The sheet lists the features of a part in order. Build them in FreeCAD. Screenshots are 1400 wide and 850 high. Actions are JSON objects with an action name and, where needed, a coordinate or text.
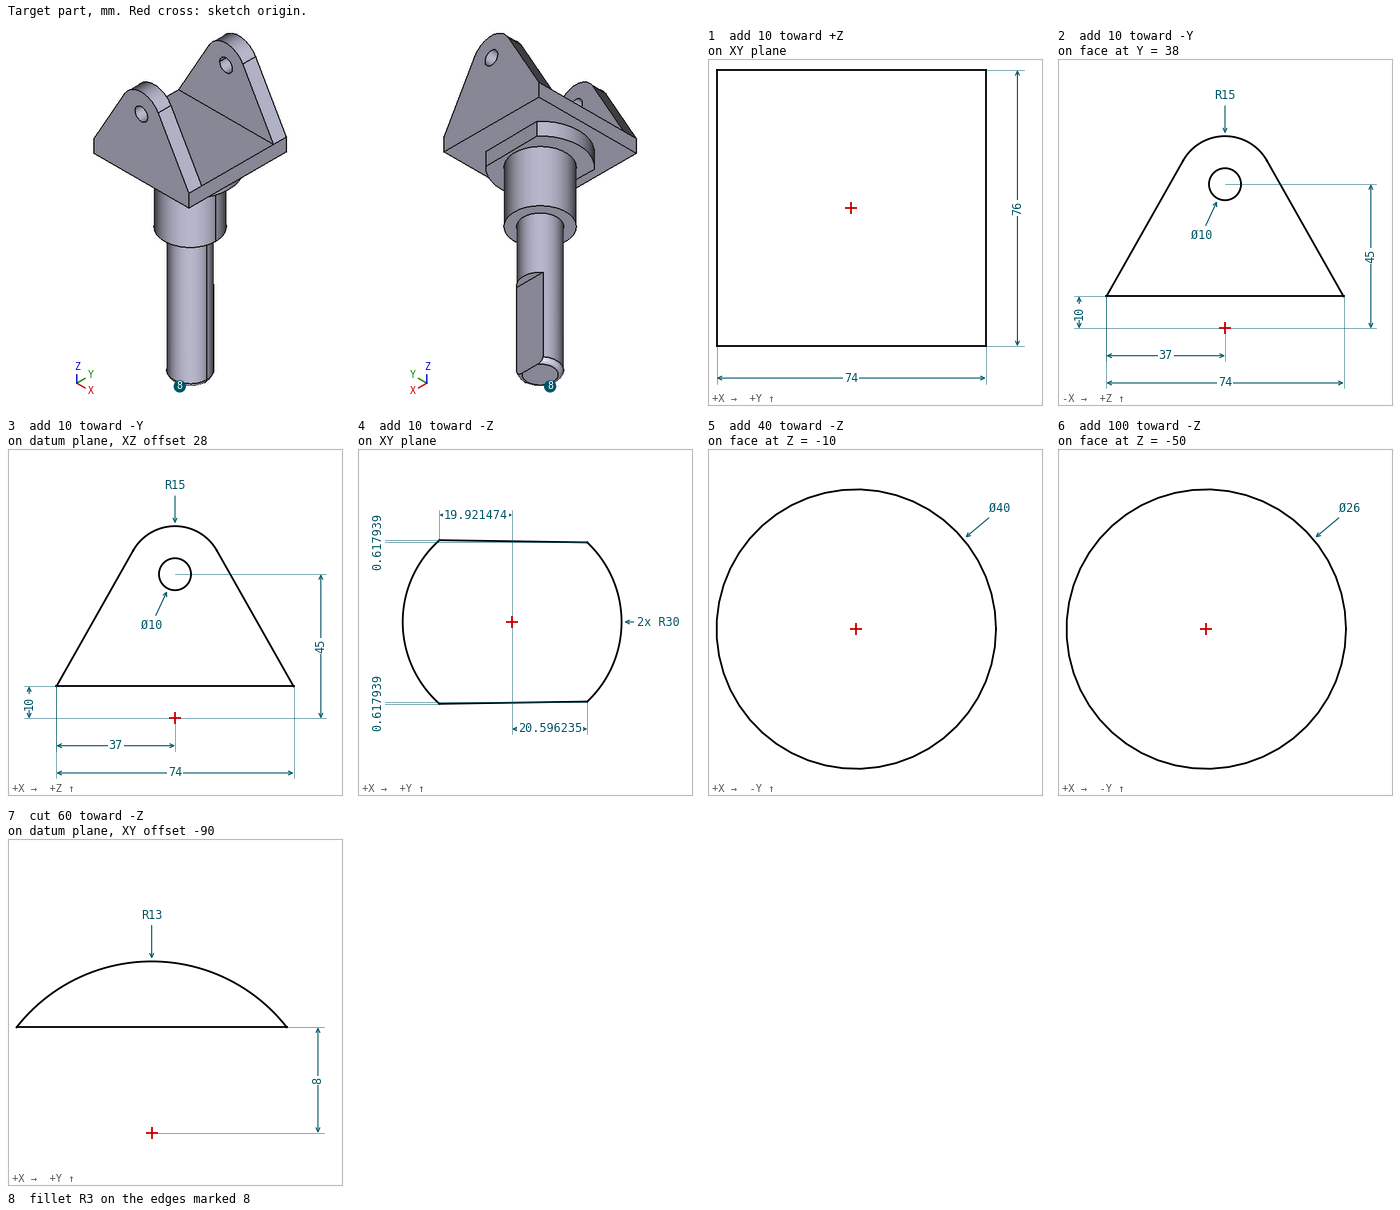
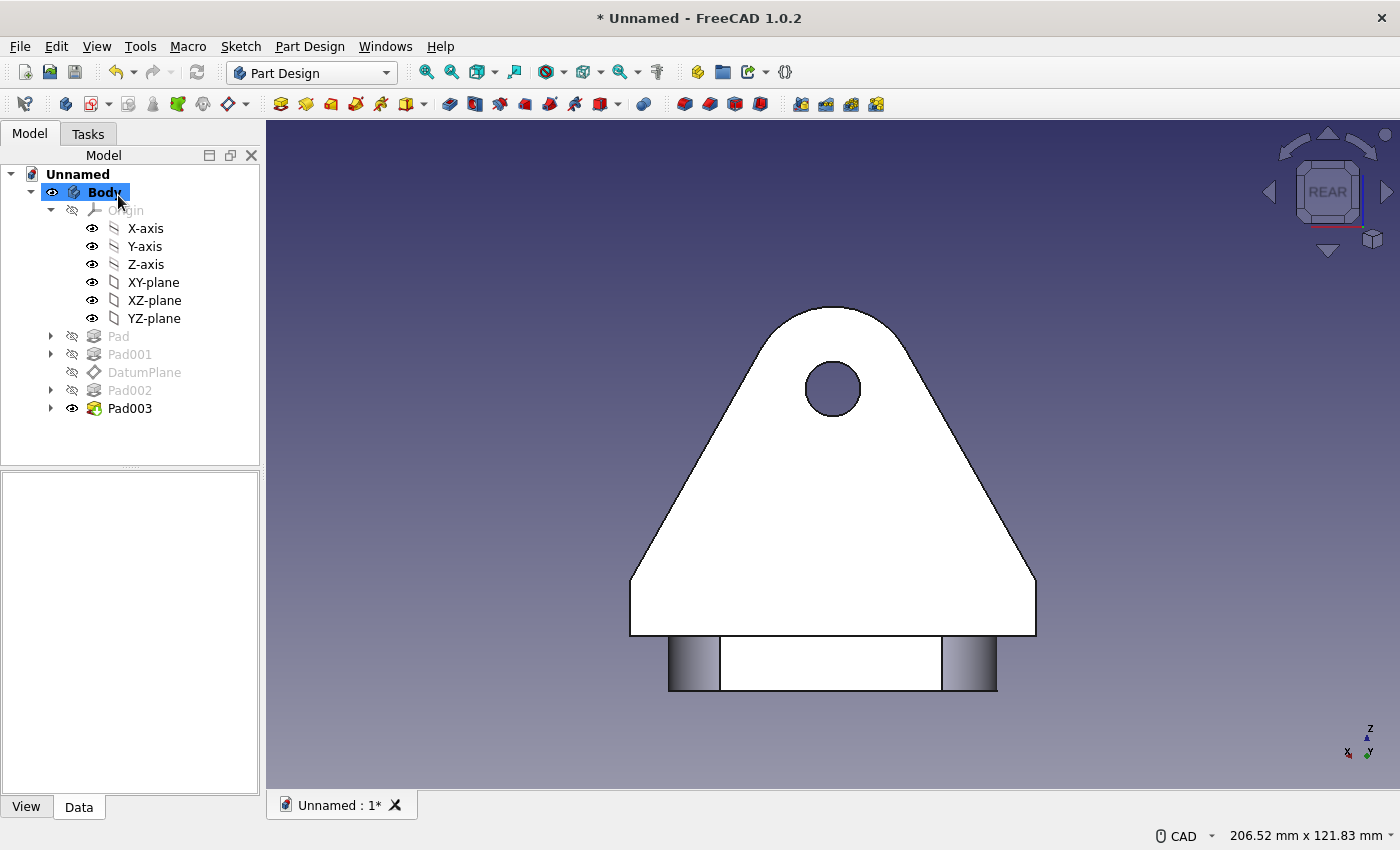
{"action": "key", "text": "5"}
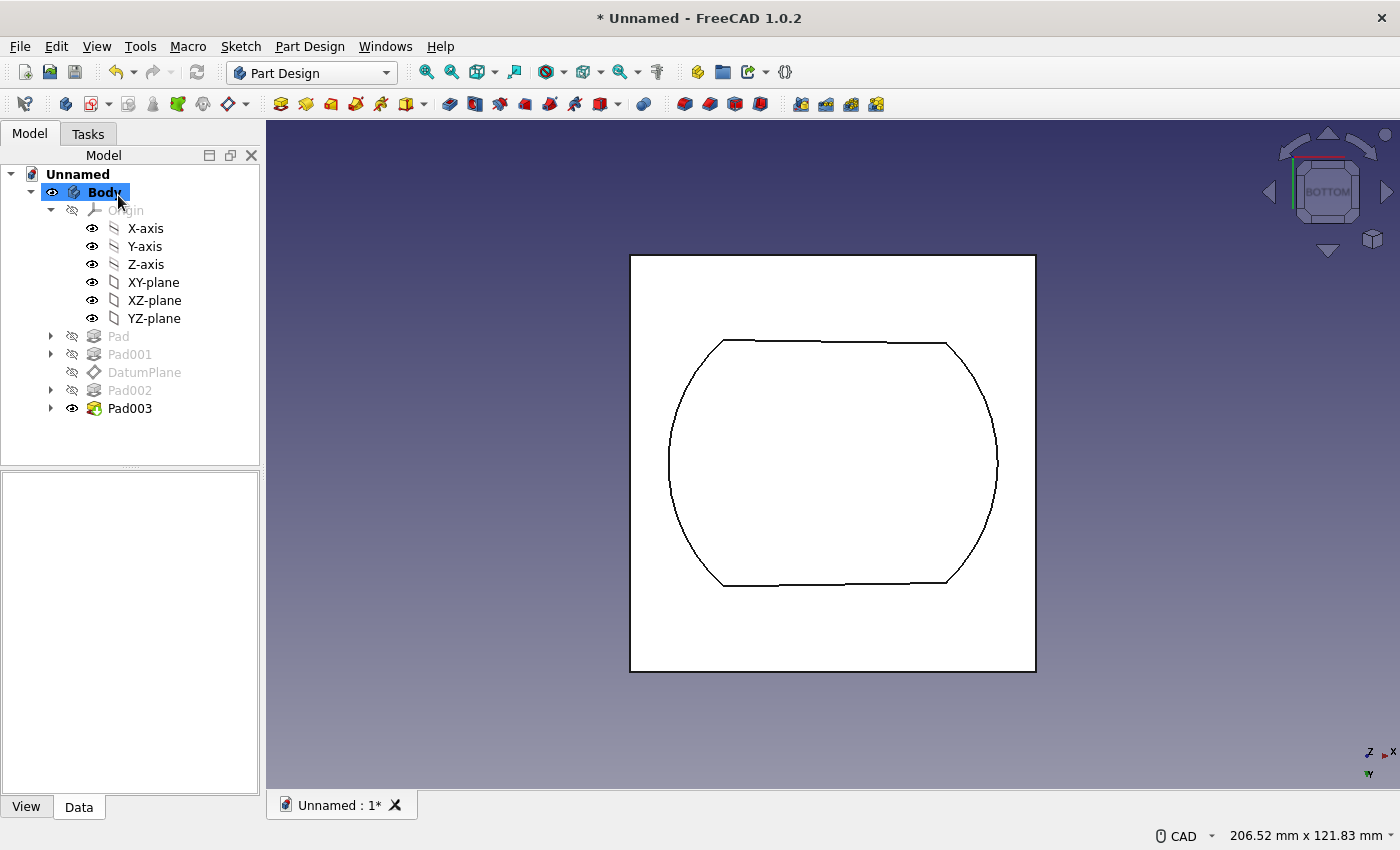
{"action": "left_click", "coordinate": [833, 462]}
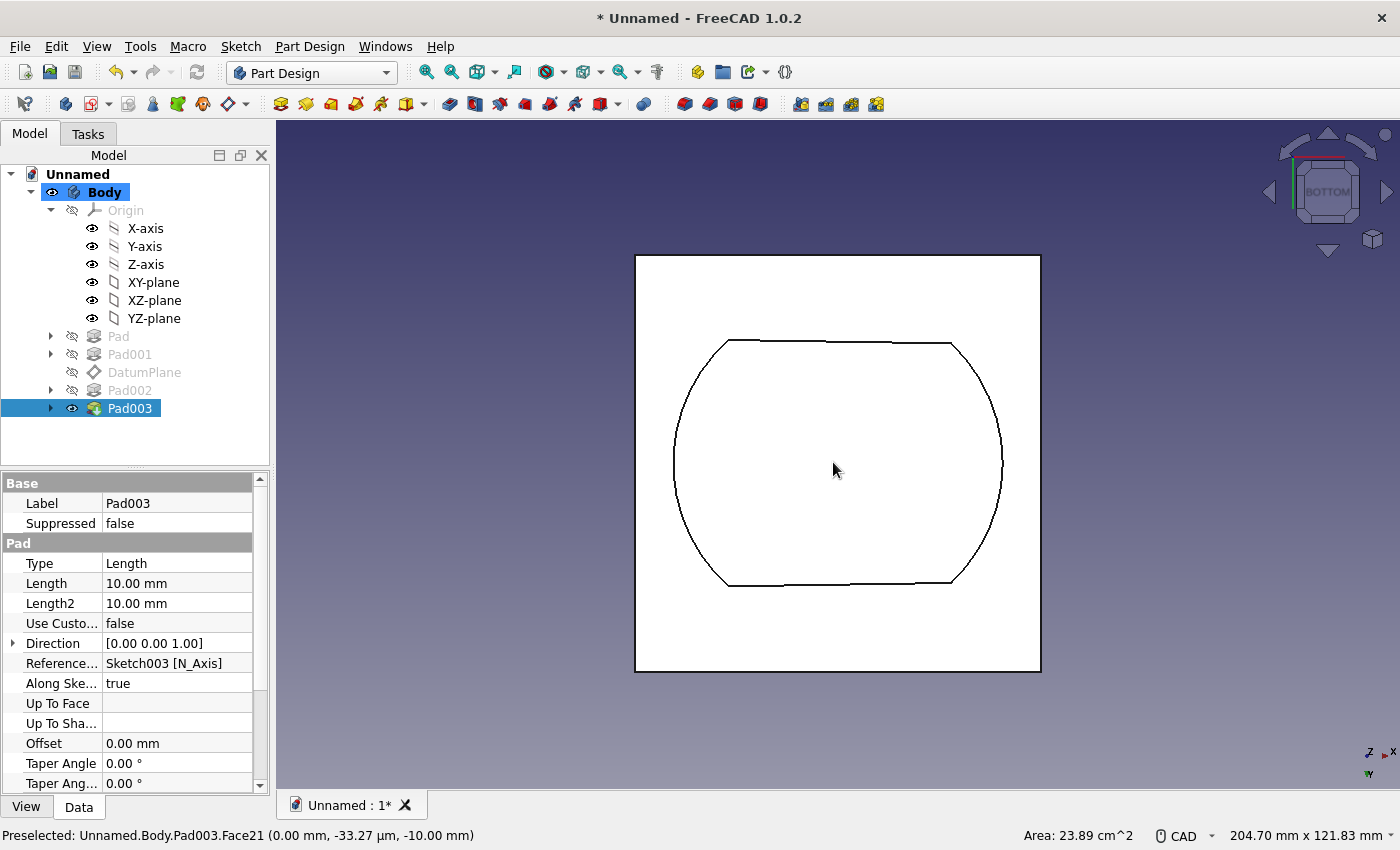
{"action": "left_click", "coordinate": [90, 104]}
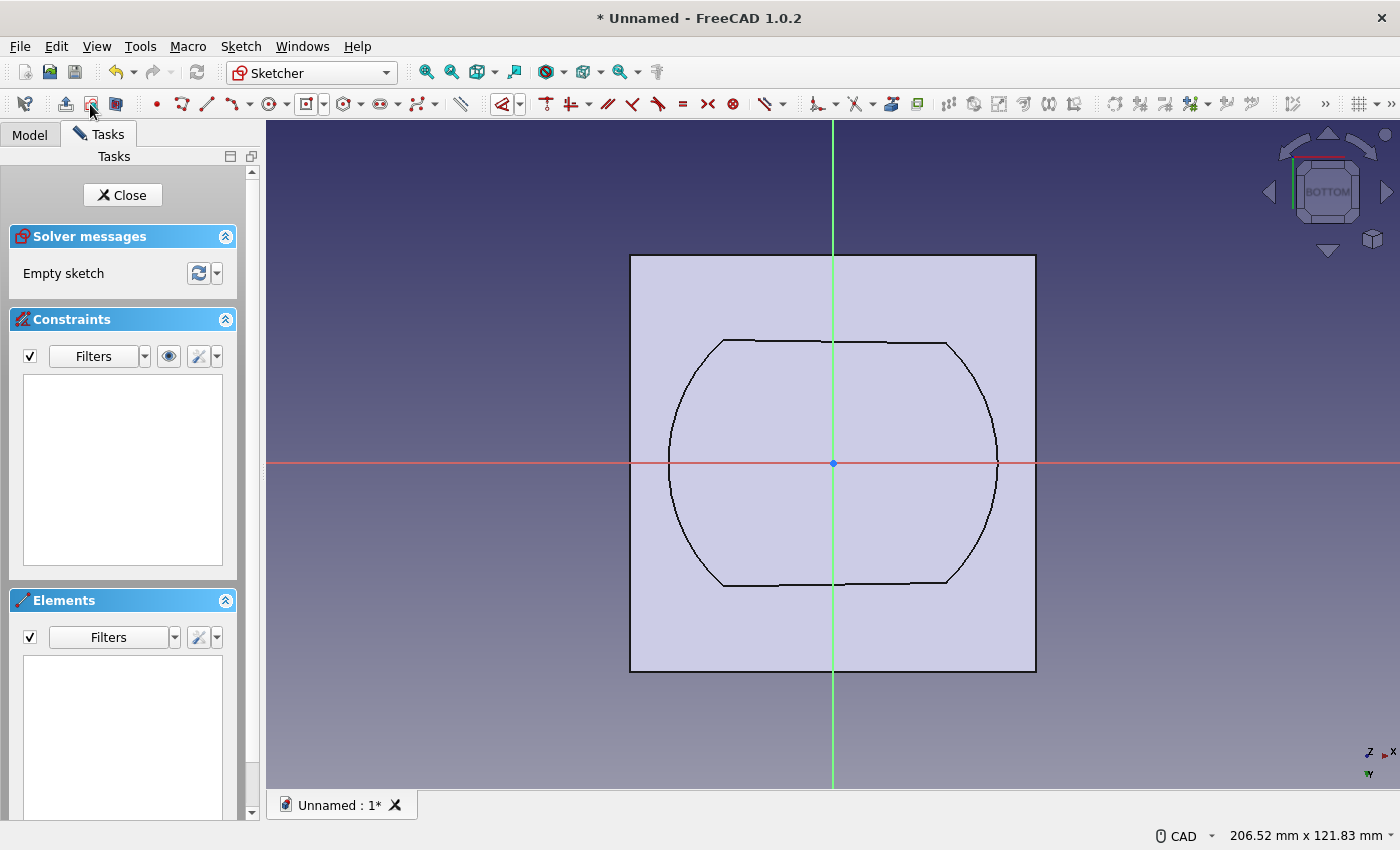
{"action": "scroll", "coordinate": [916, 474], "scroll_direction": "up", "scroll_amount": 3}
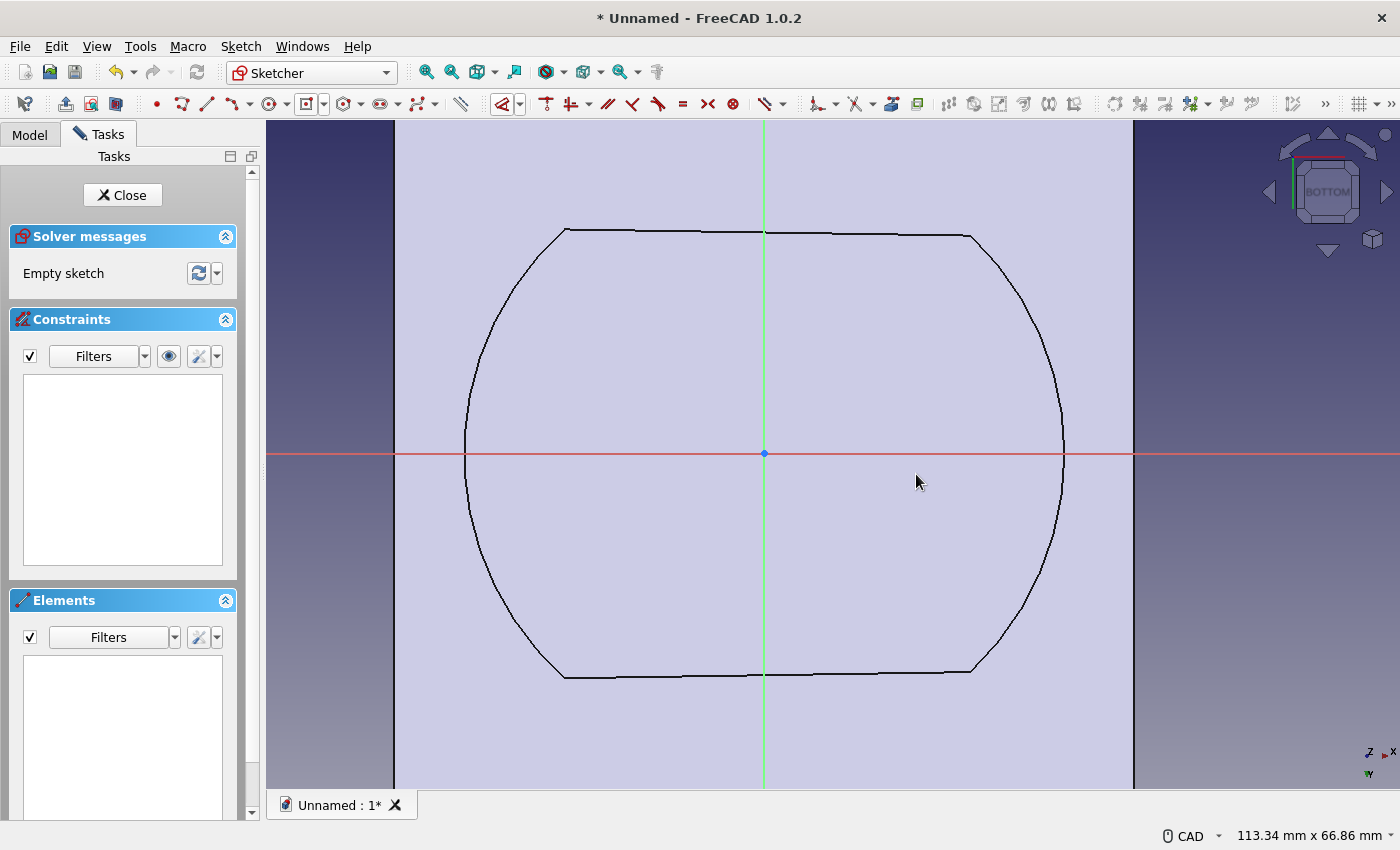
{"action": "key", "text": "g c"}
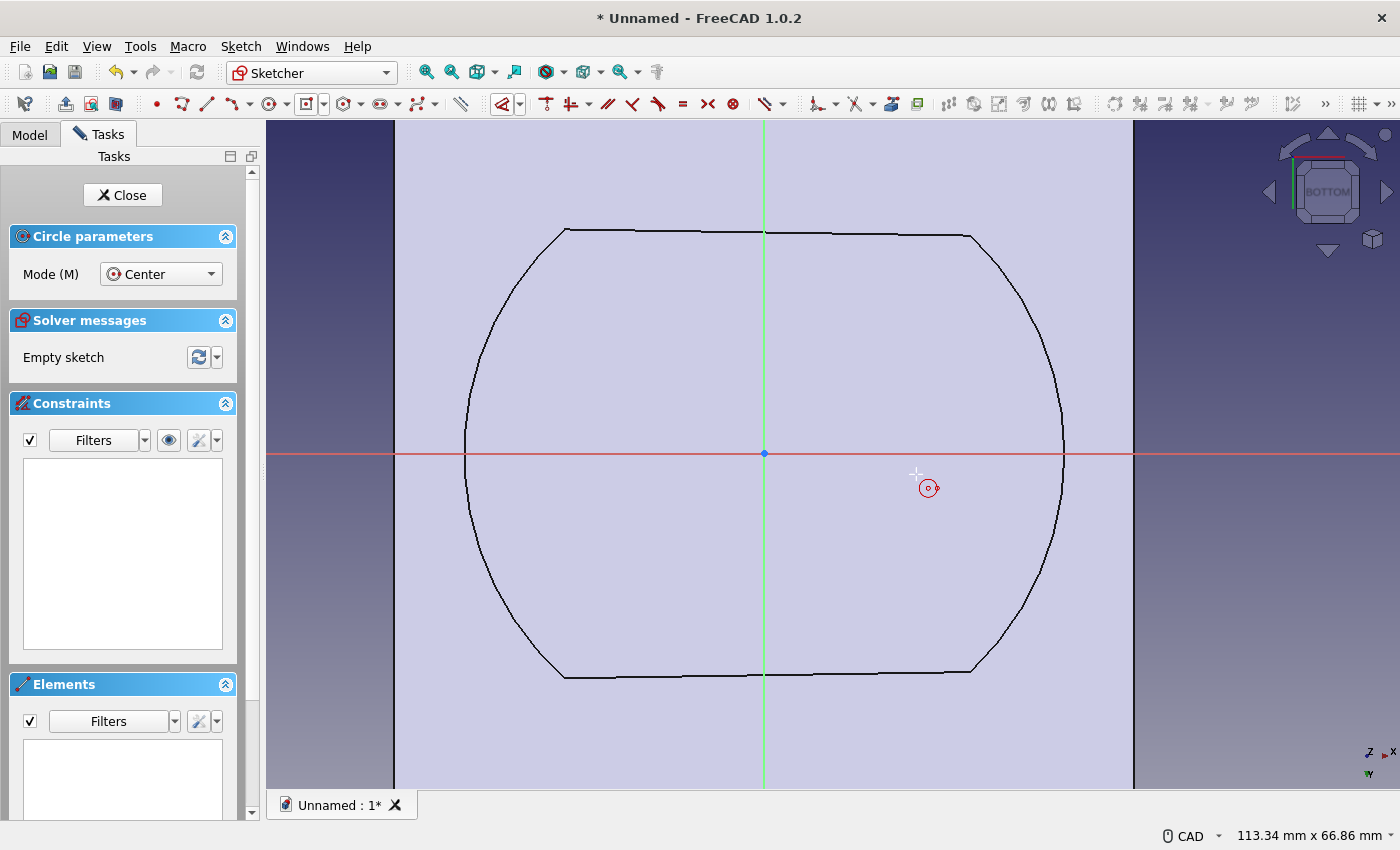
{"action": "left_click", "coordinate": [764, 454]}
{"action": "left_click", "coordinate": [906, 312]}
{"action": "key", "text": "Escape"}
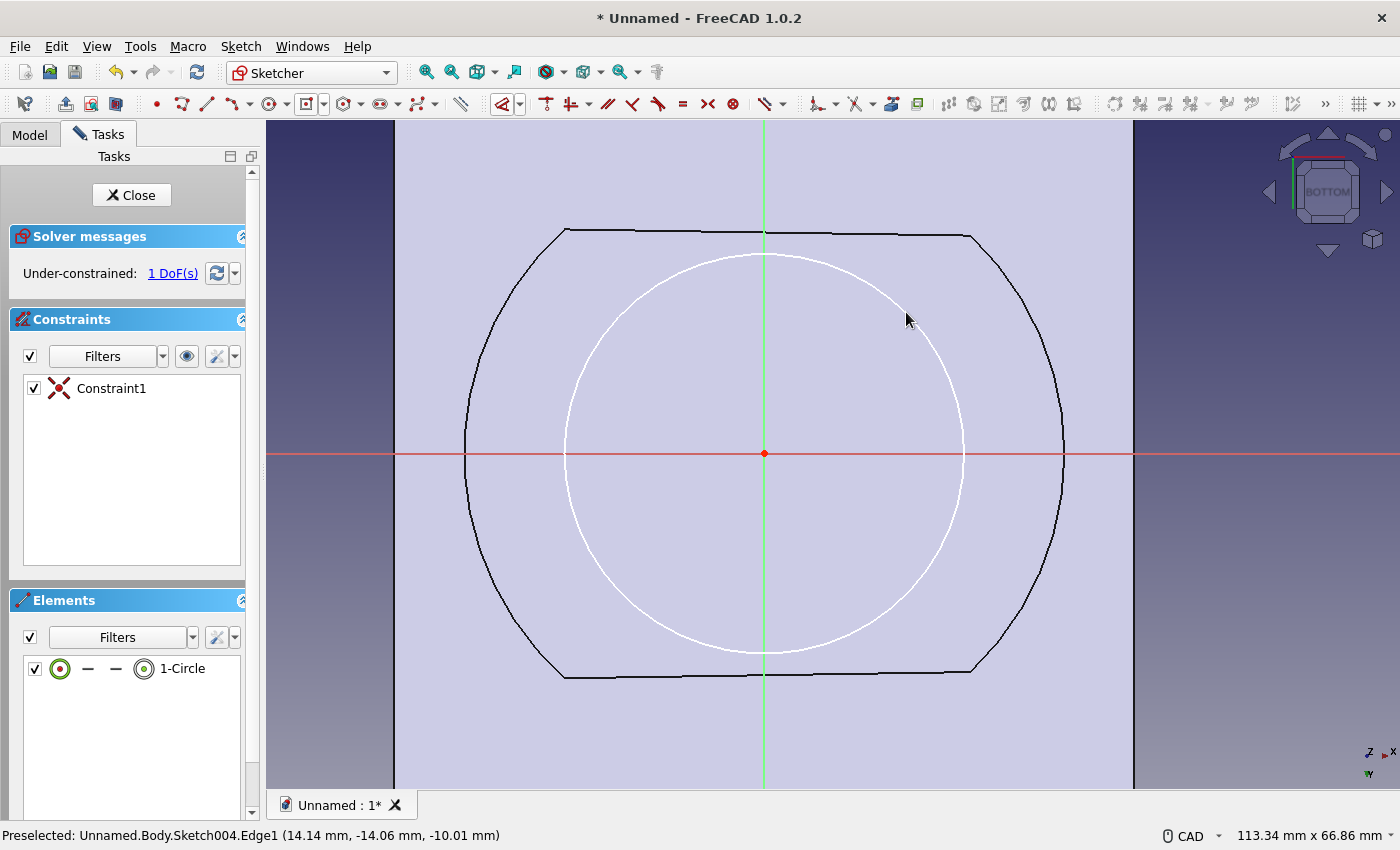
{"action": "left_click", "coordinate": [905, 312]}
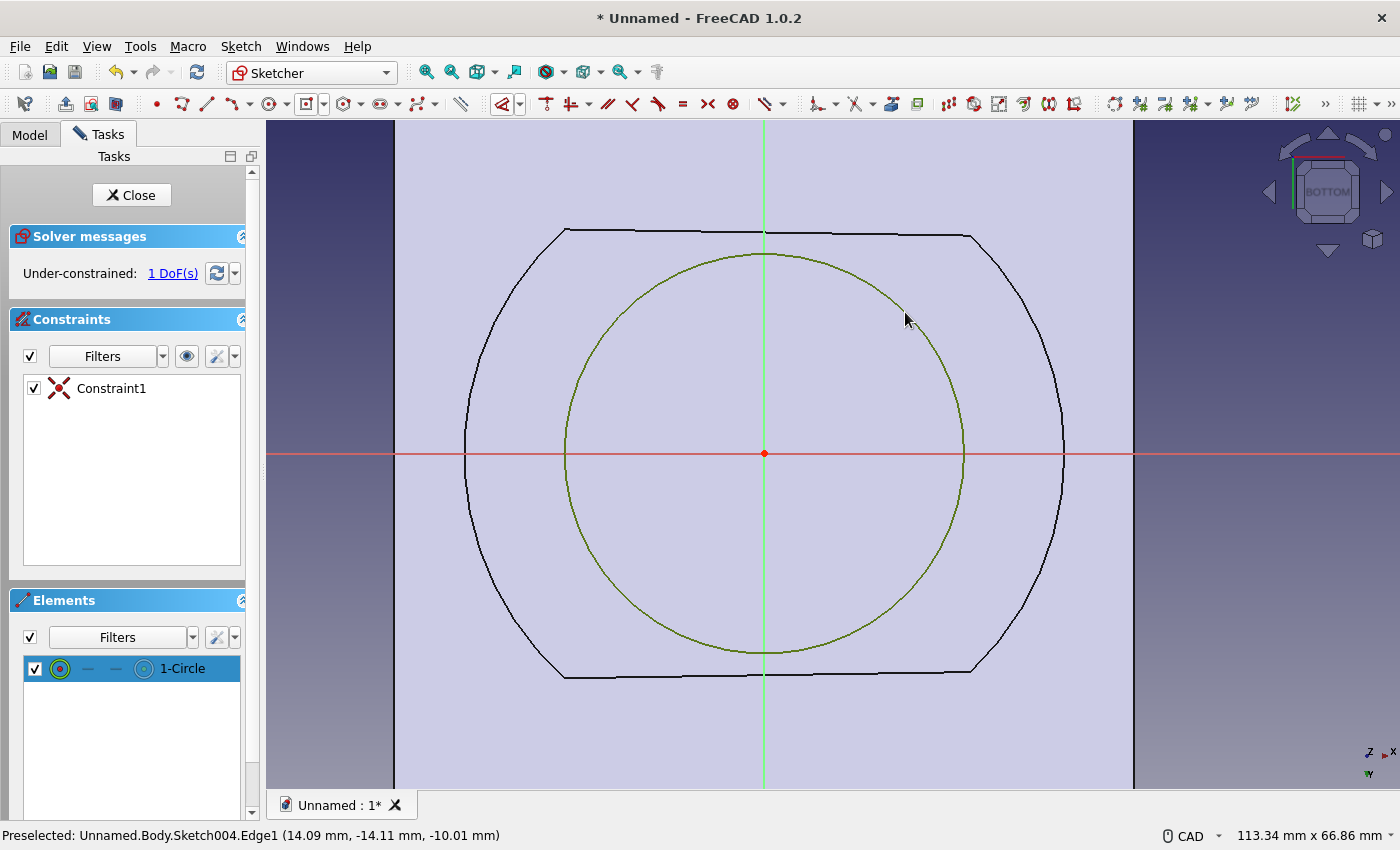
{"action": "key", "text": "k o"}